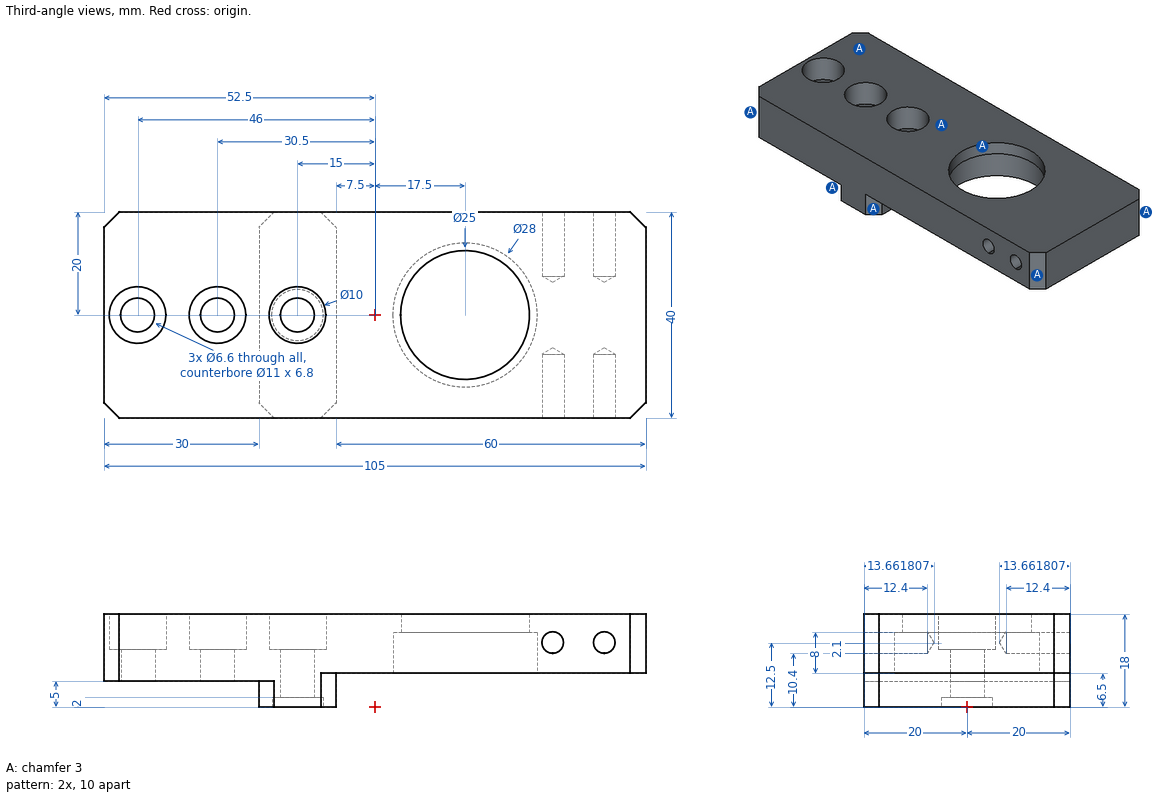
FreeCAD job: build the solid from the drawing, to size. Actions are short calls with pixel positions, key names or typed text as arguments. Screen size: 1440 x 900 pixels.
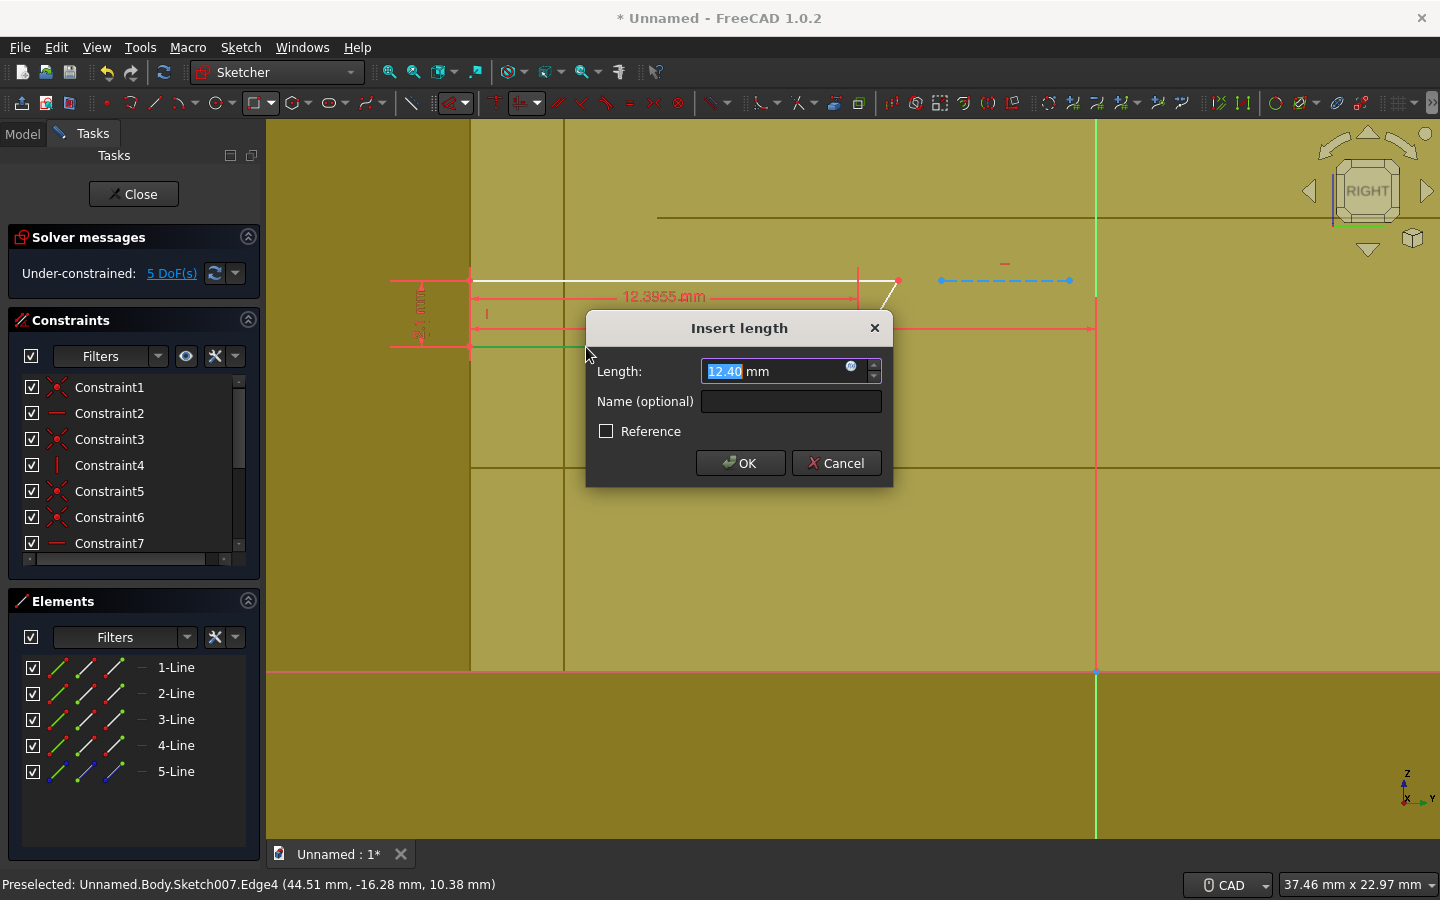
text(12.4)
key(Return)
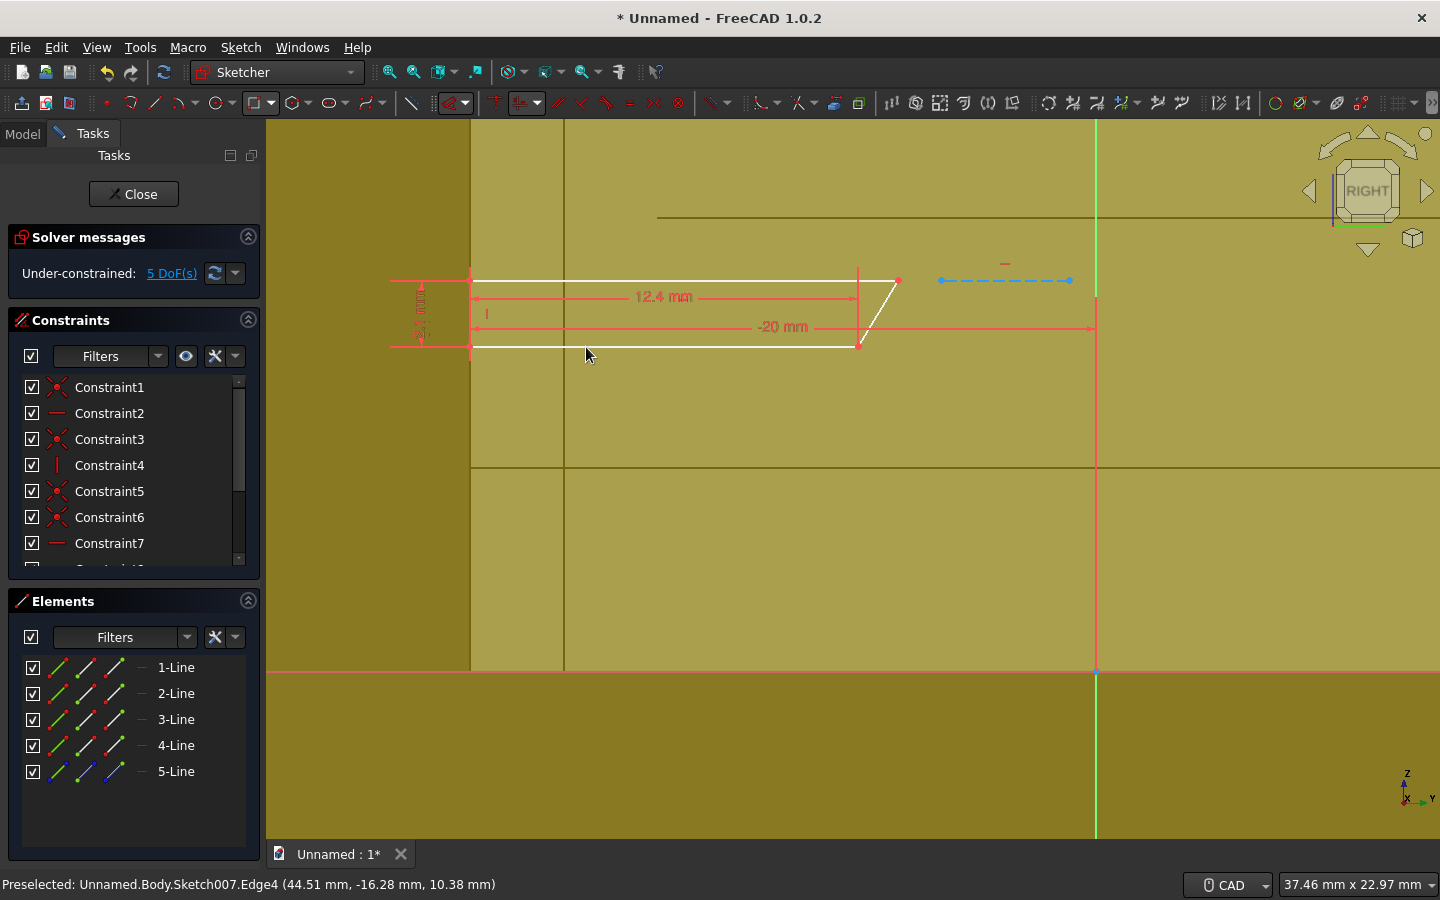
click(858, 347)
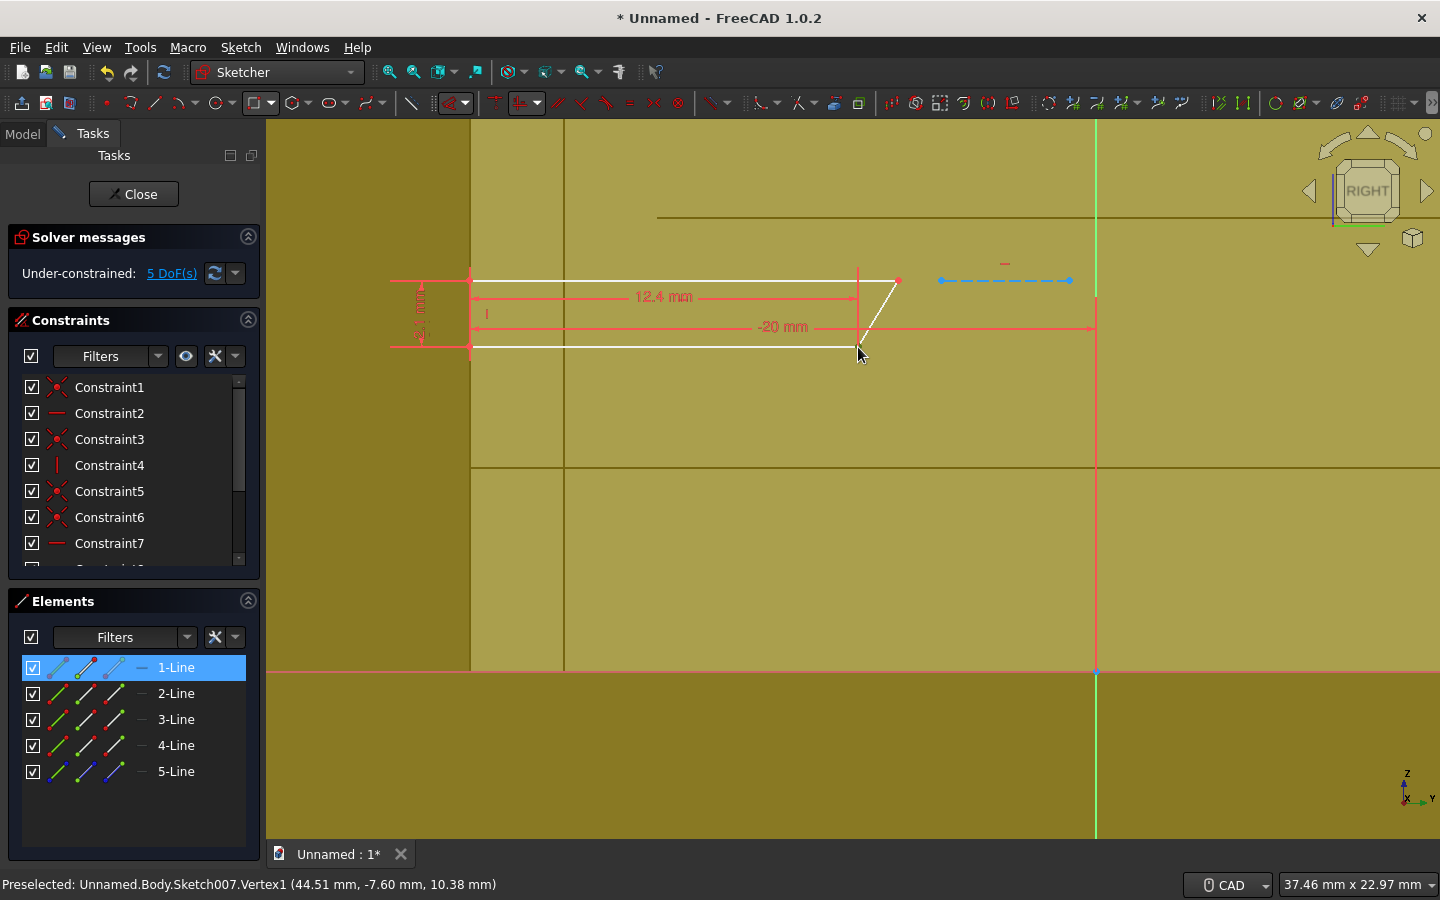
click(468, 104)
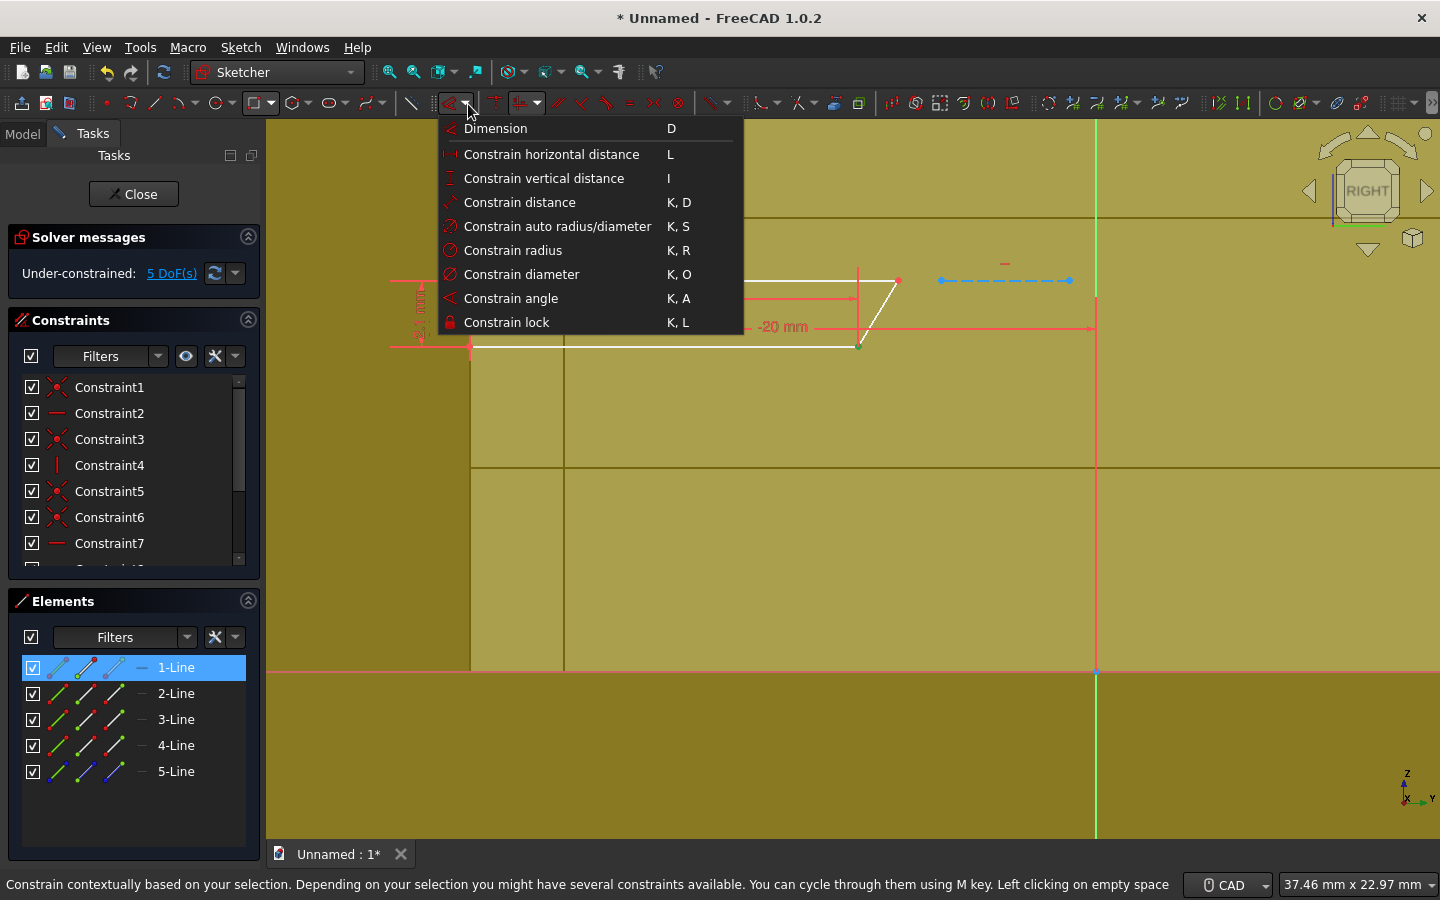
click(591, 178)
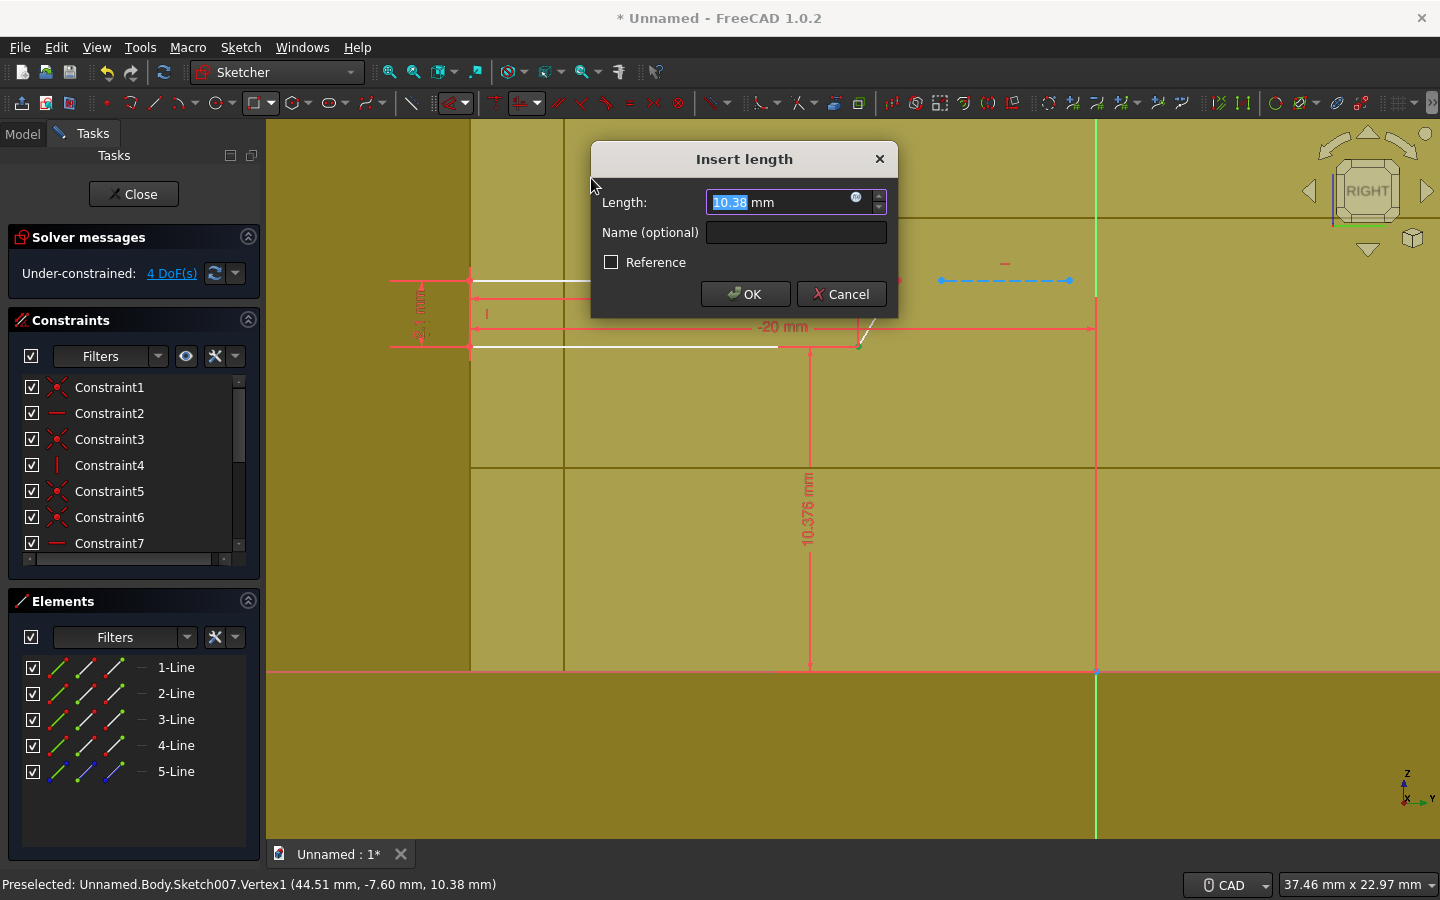
text(10.4)
key(Return)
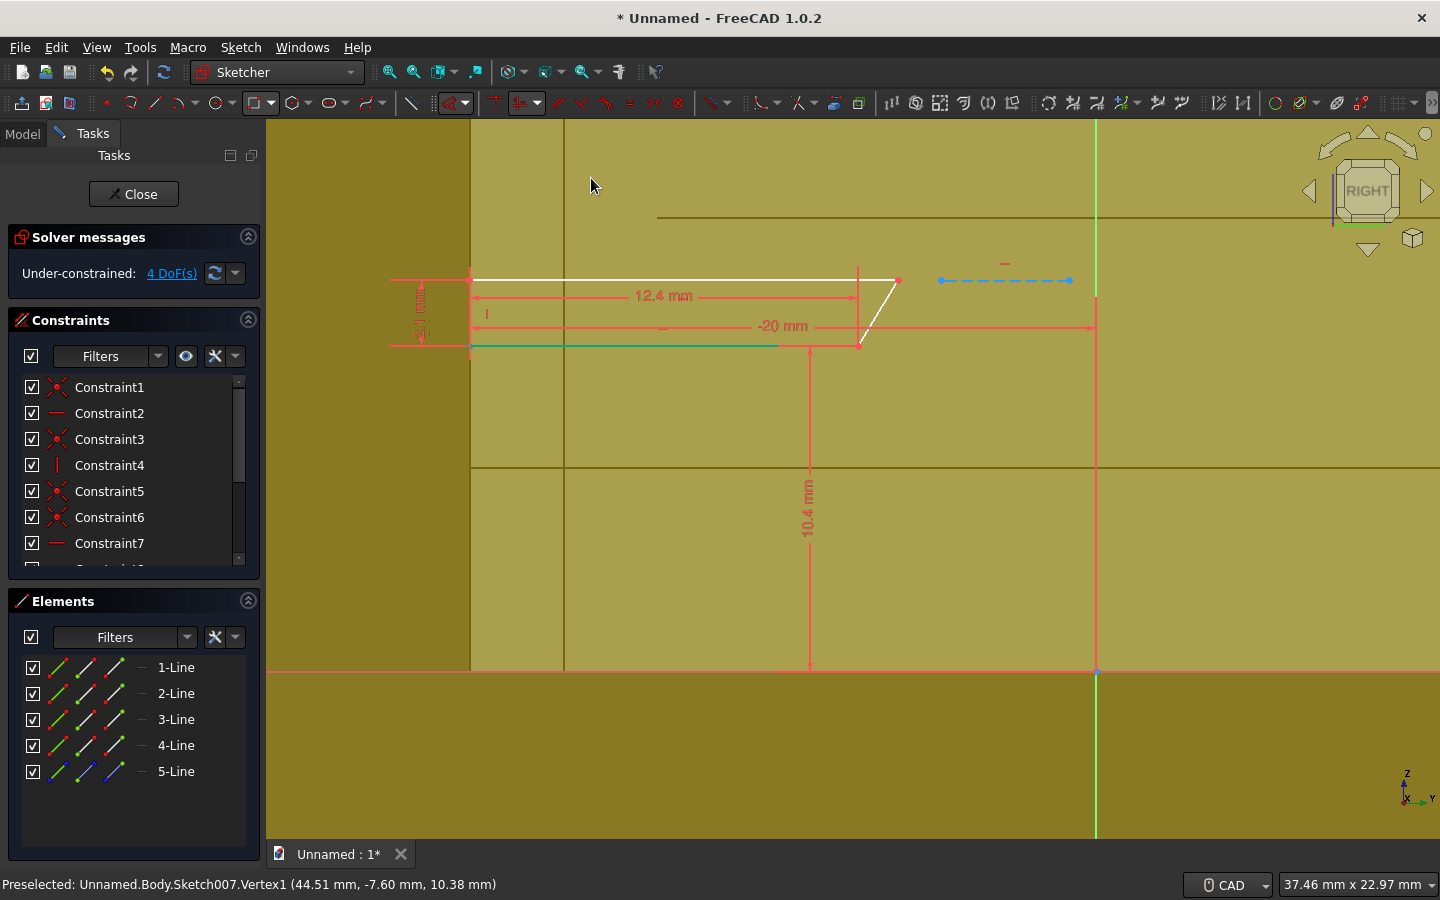
click(941, 281)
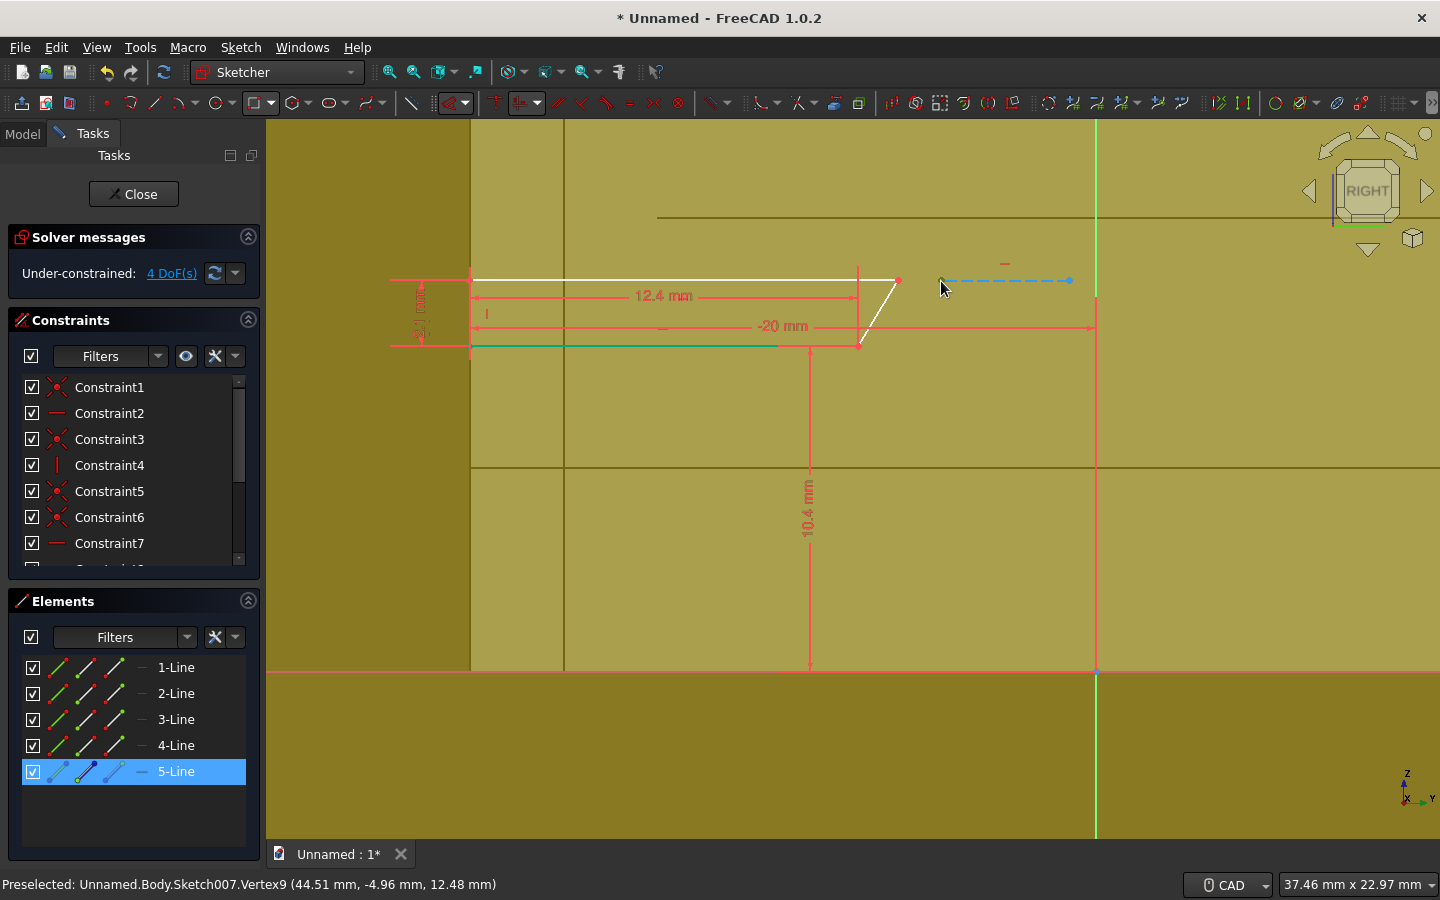
click(468, 104)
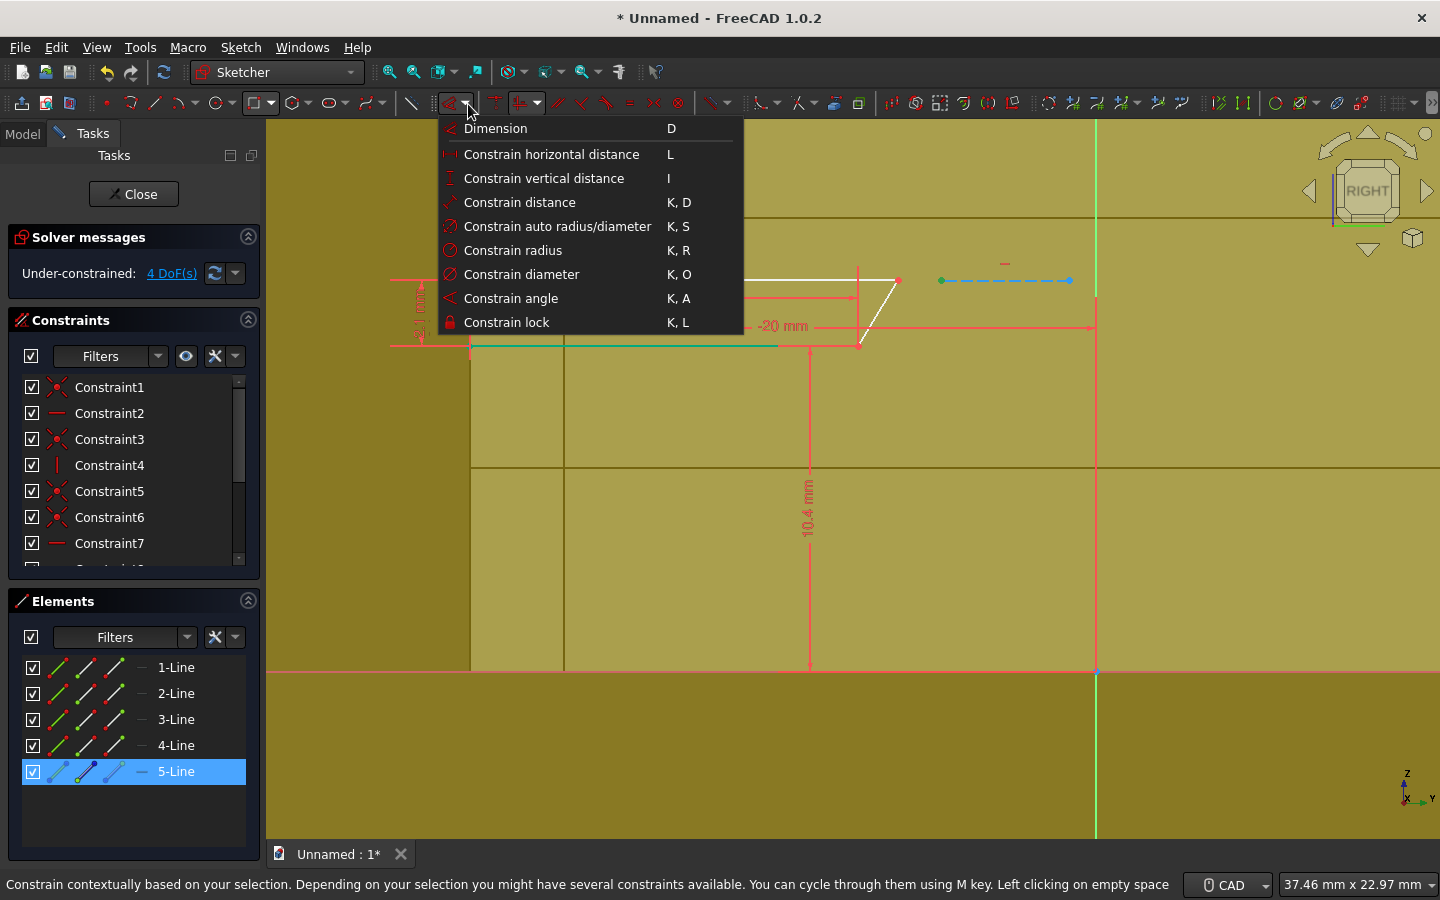
click(591, 178)